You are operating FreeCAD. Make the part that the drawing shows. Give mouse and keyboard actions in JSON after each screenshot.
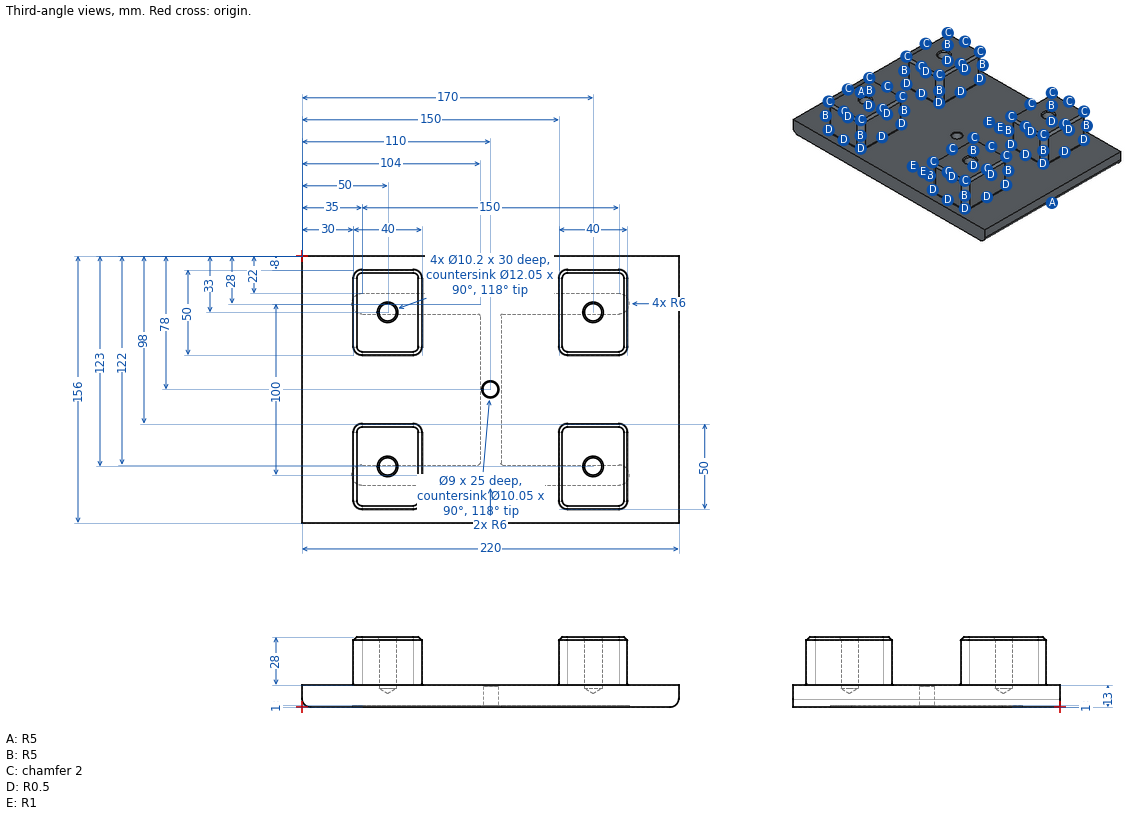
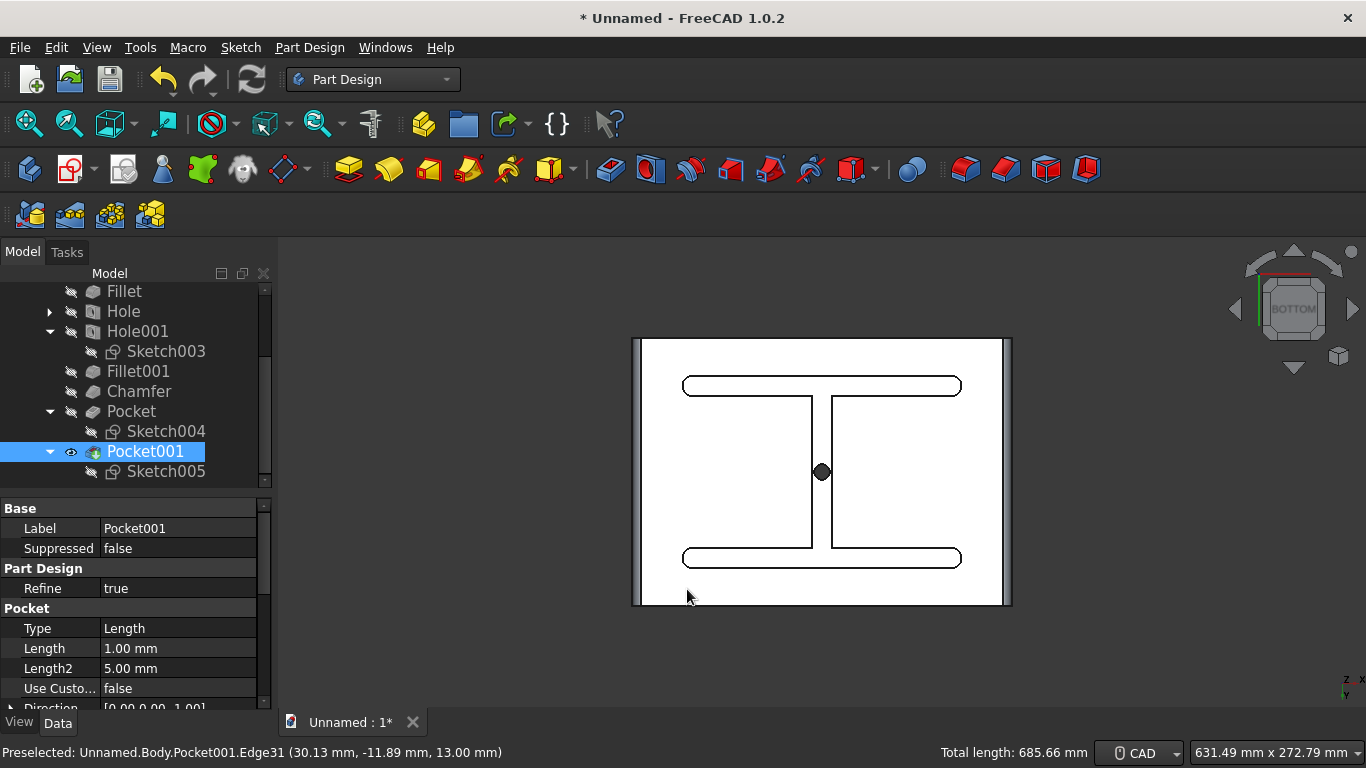
{"action": "left_click", "coordinate": [966, 170]}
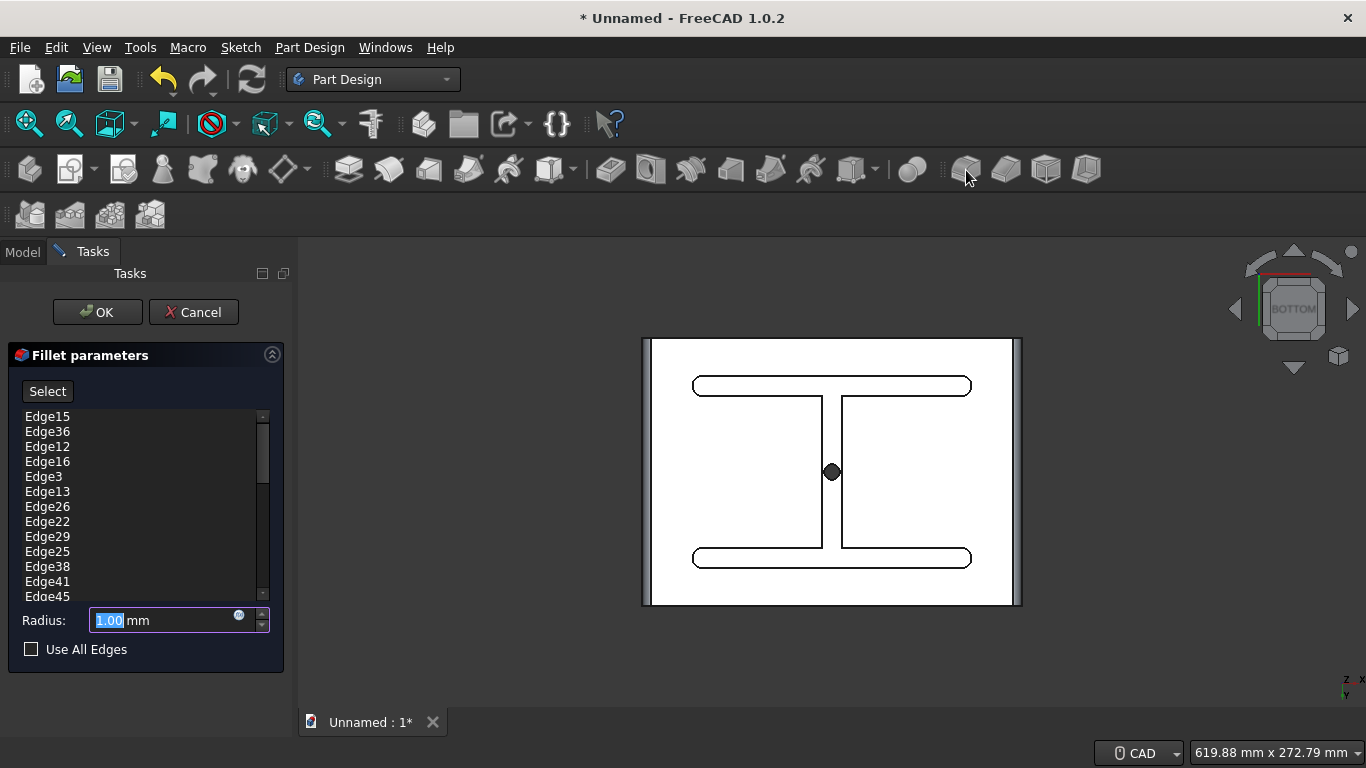
{"action": "type", "text": "0.5"}
{"action": "key", "text": "Tab"}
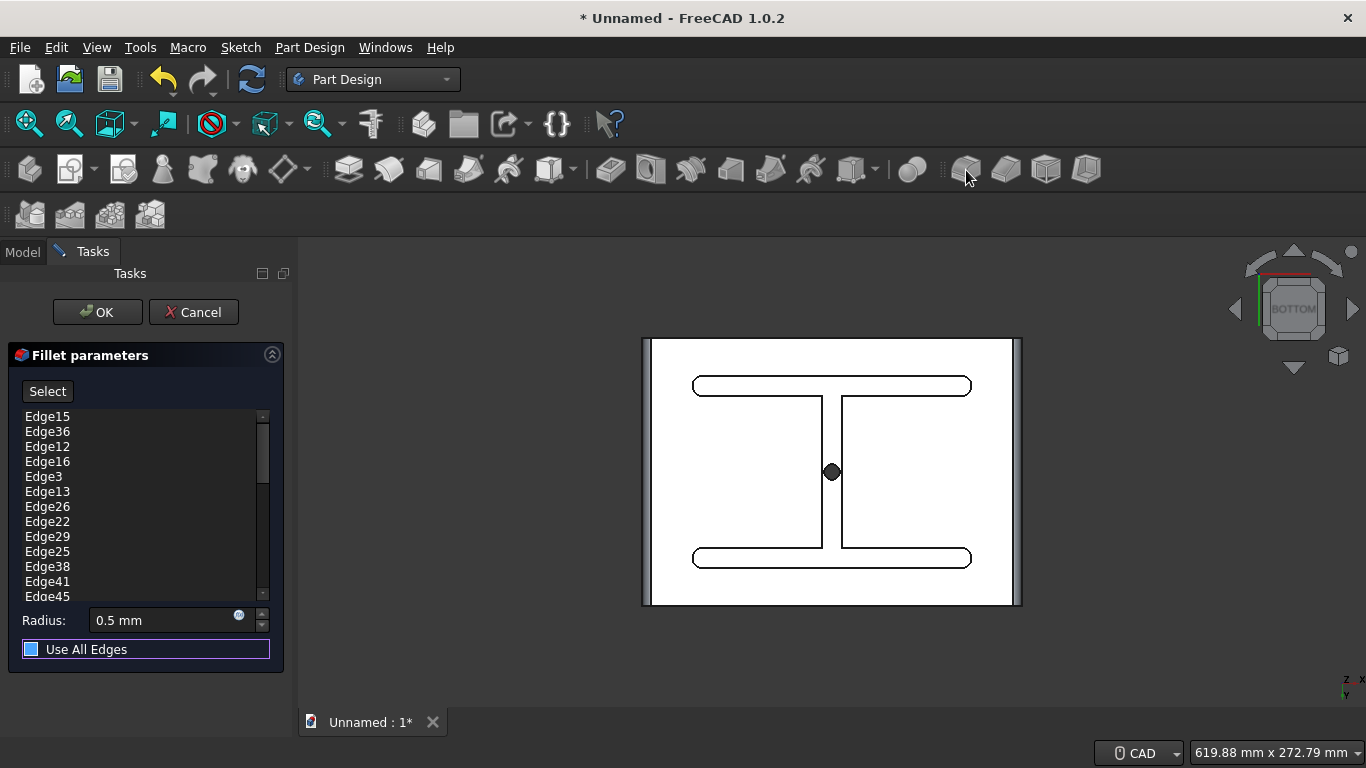
{"action": "left_click", "coordinate": [98, 312]}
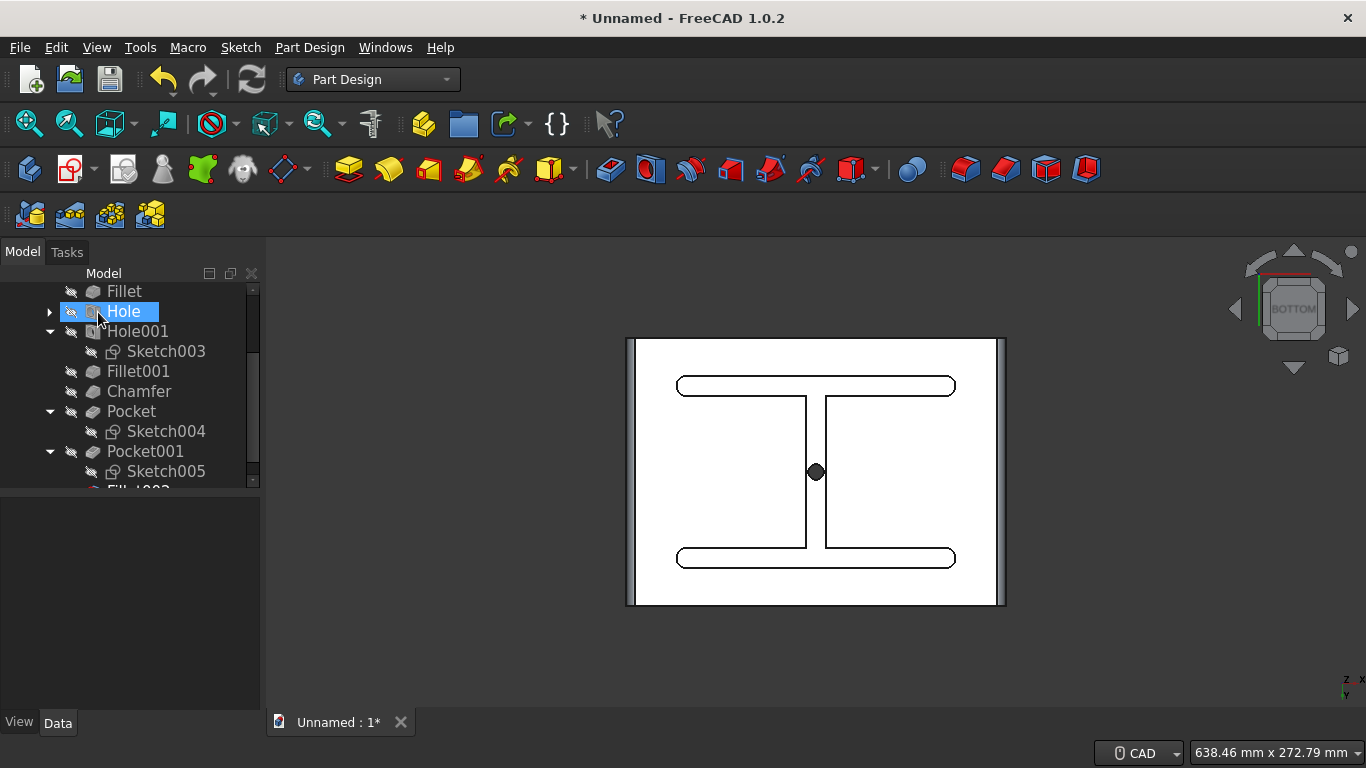
{"action": "scroll", "coordinate": [806, 395], "scroll_direction": "up", "scroll_amount": 15}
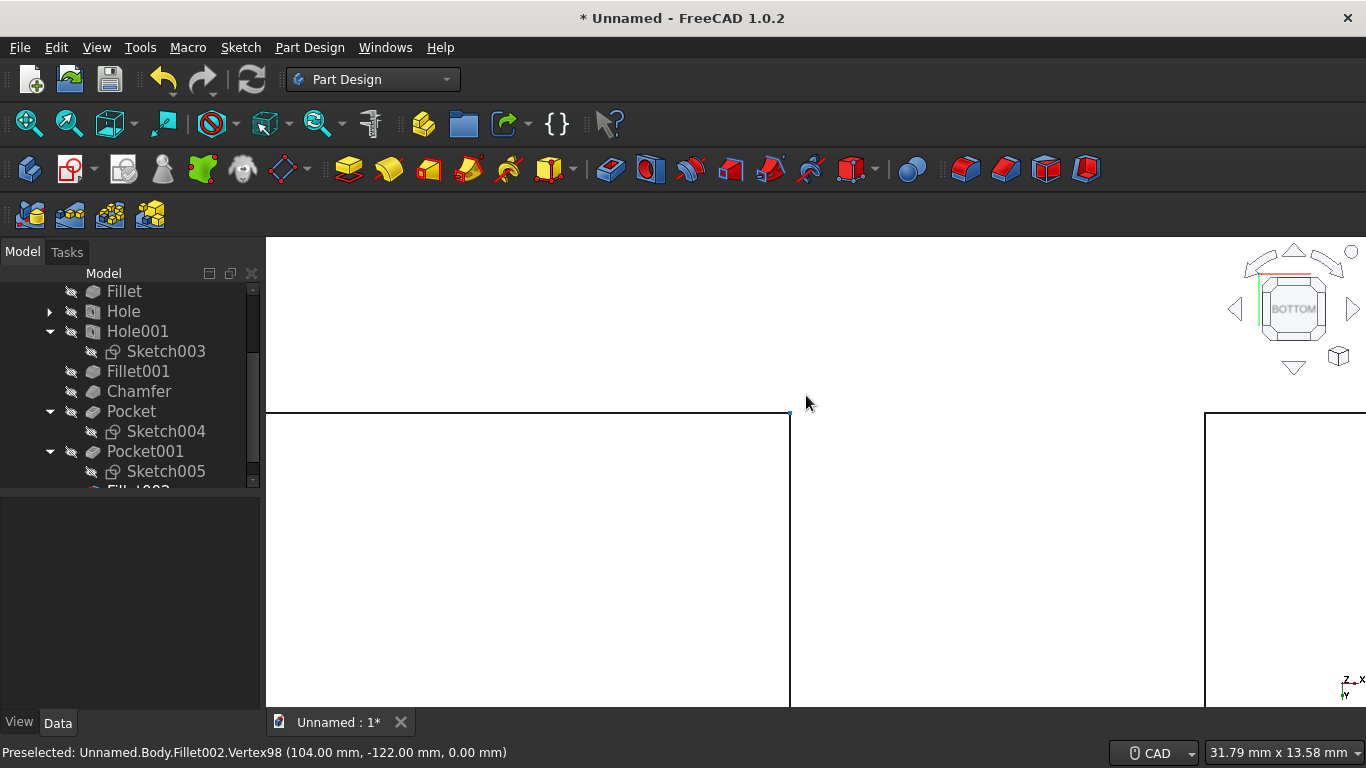
{"action": "key", "text": "v f"}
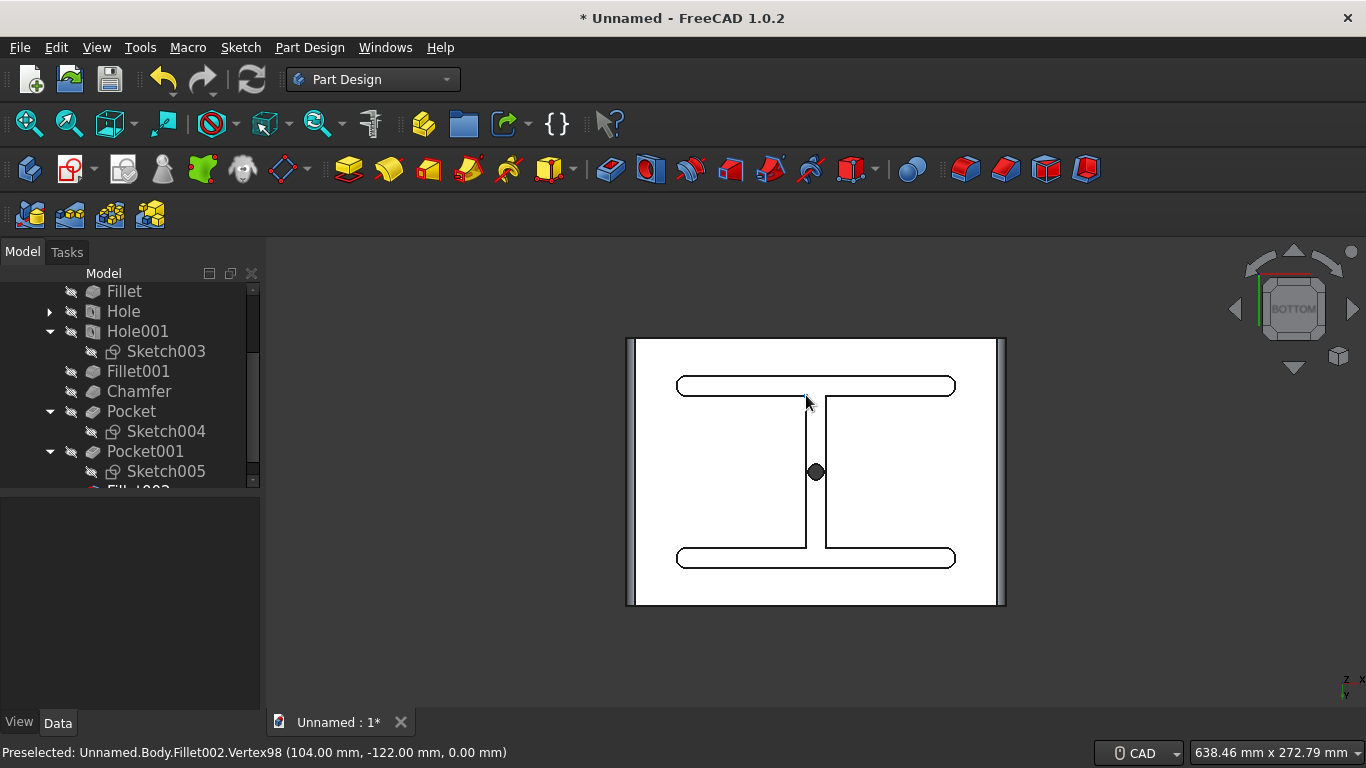
{"action": "key", "text": "0"}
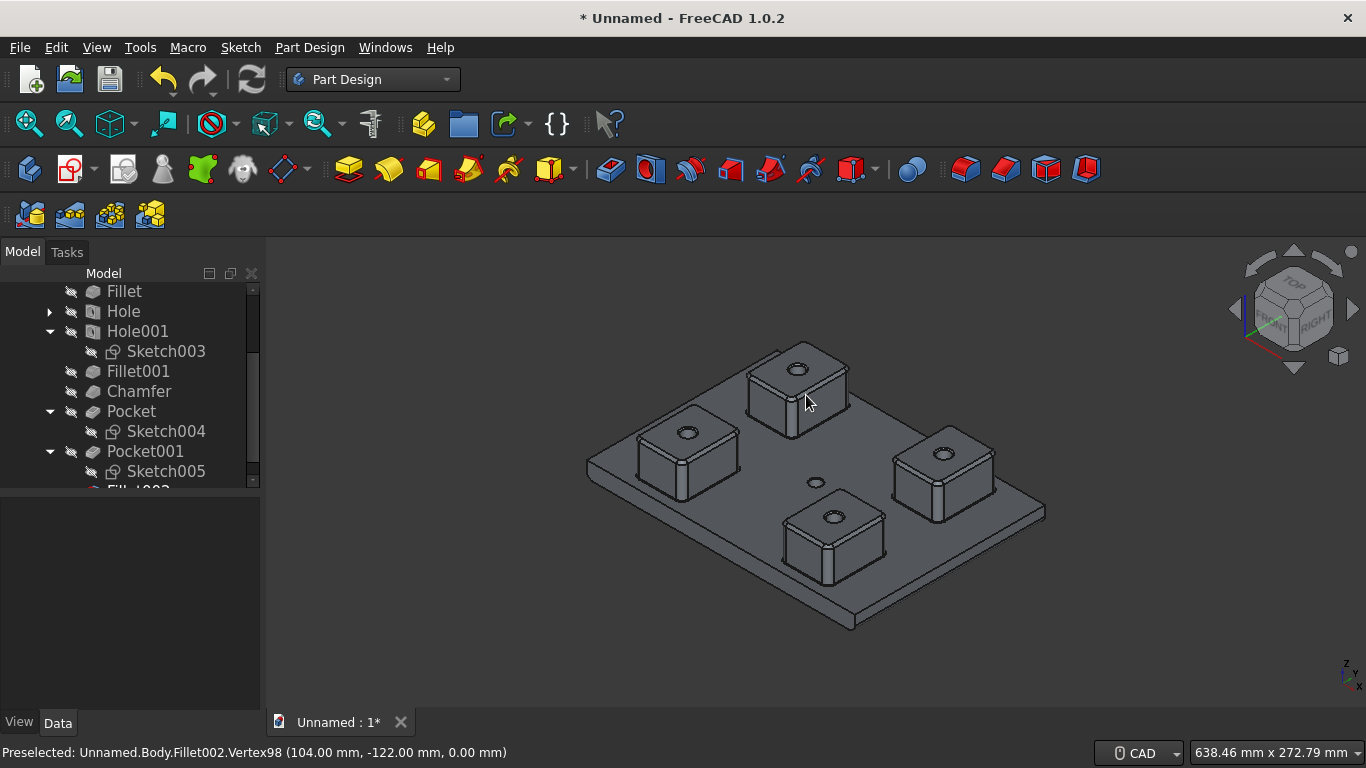
{"action": "scroll", "coordinate": [755, 526], "scroll_direction": "up", "scroll_amount": 15}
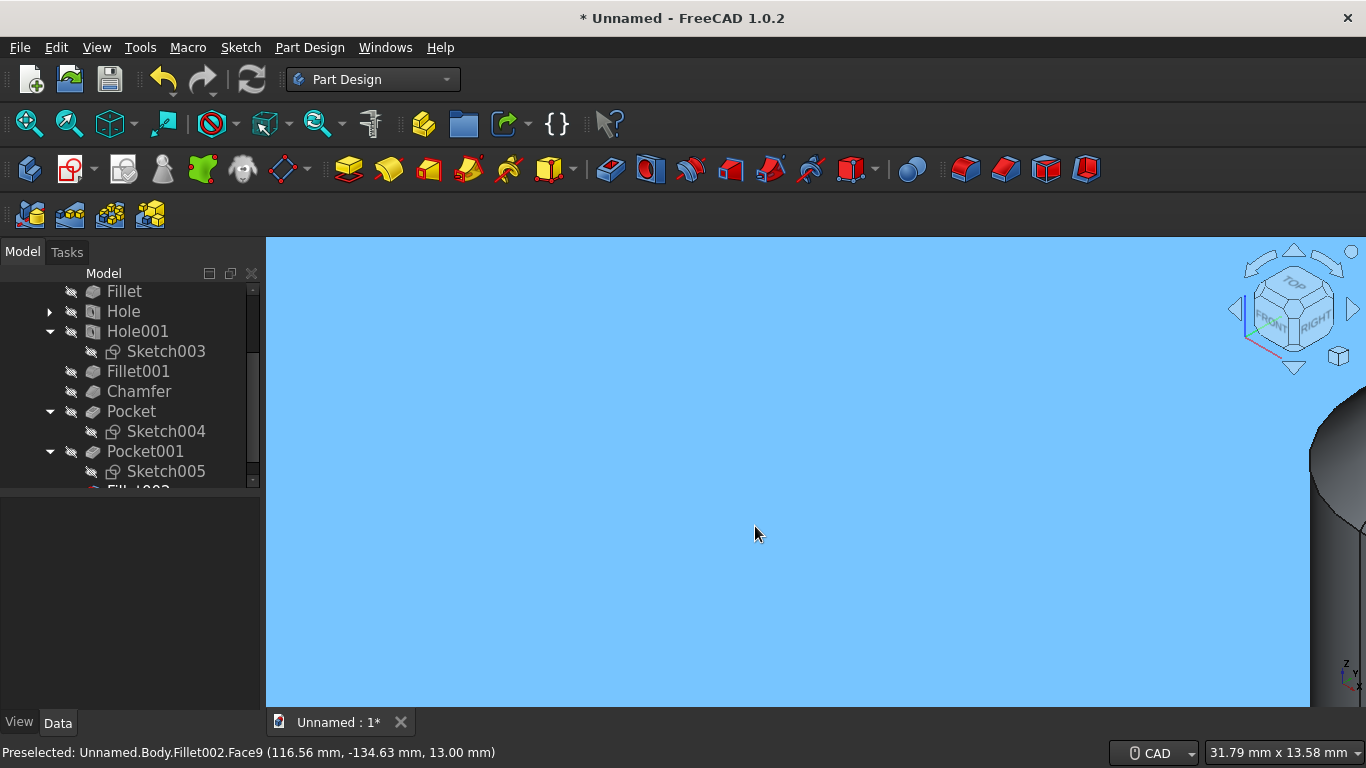
{"action": "left_click", "coordinate": [30, 124]}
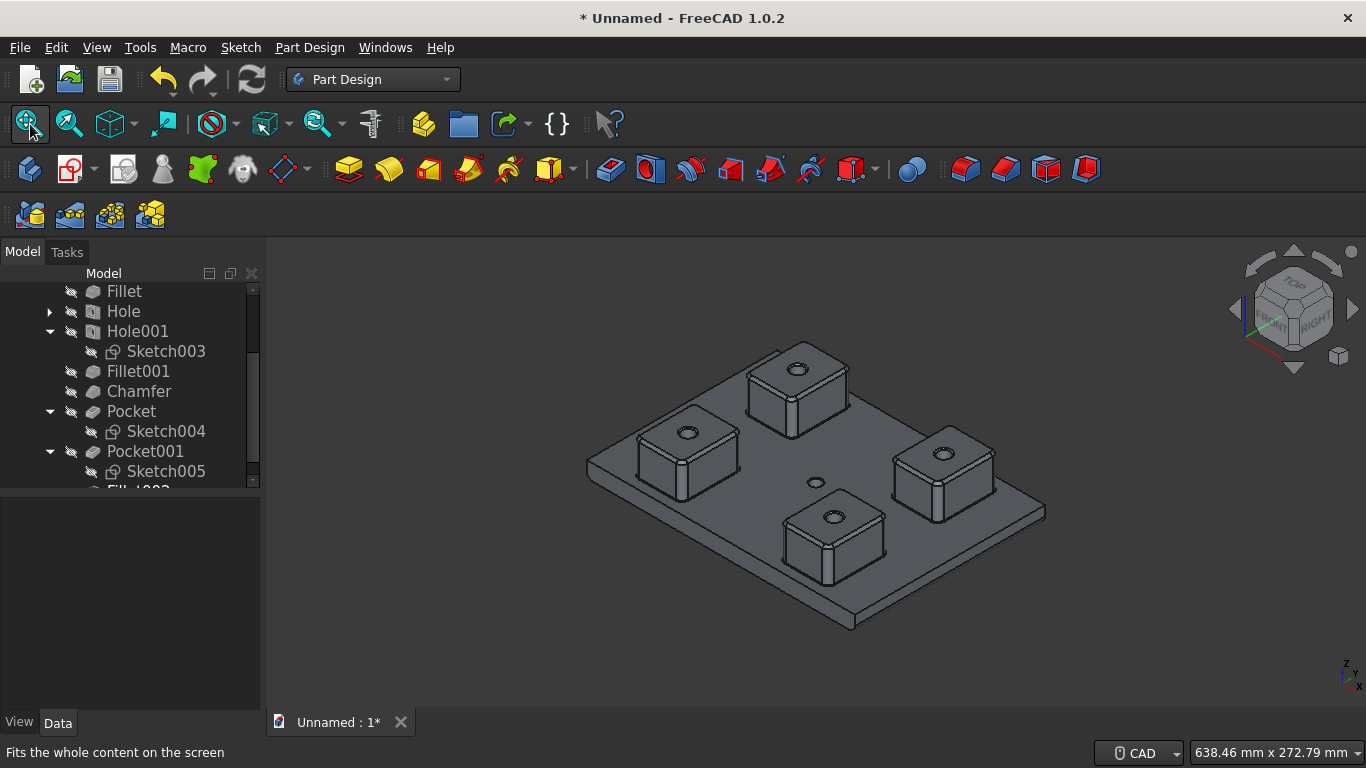
{"action": "key", "text": "2"}